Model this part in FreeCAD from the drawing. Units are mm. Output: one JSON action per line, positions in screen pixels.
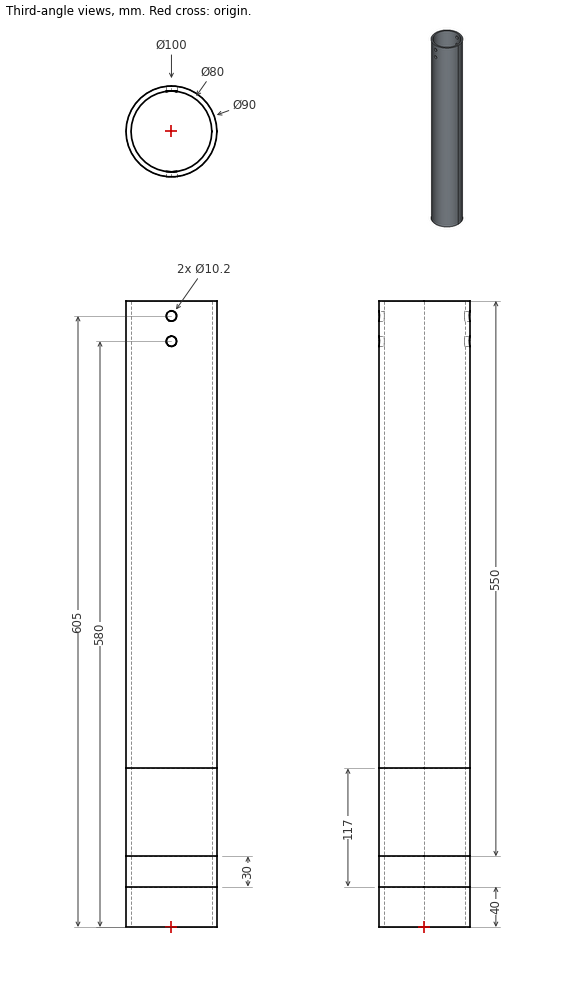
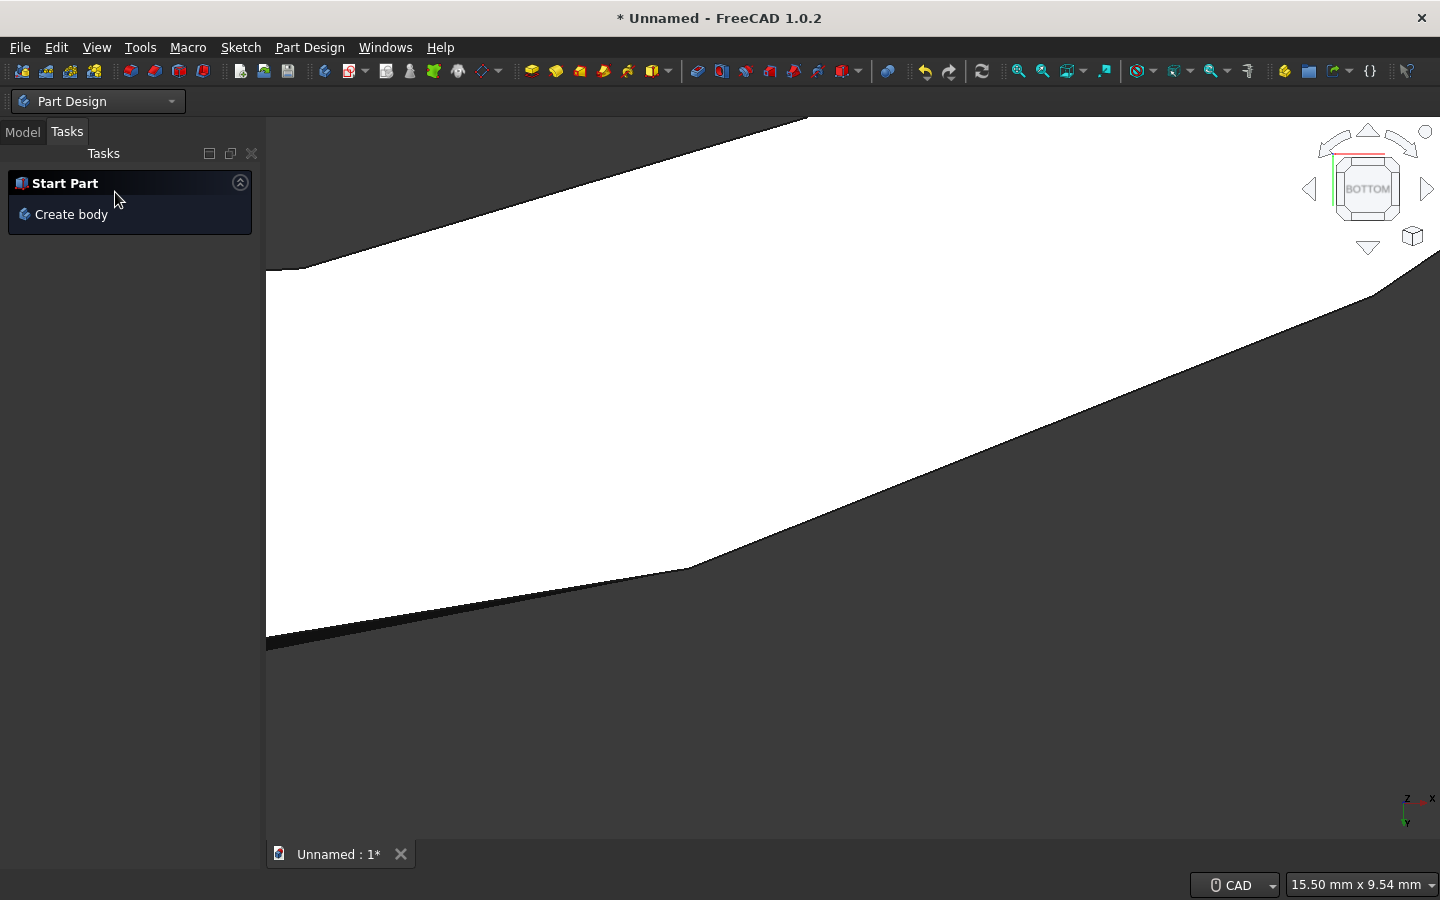
{"action": "key", "text": "0"}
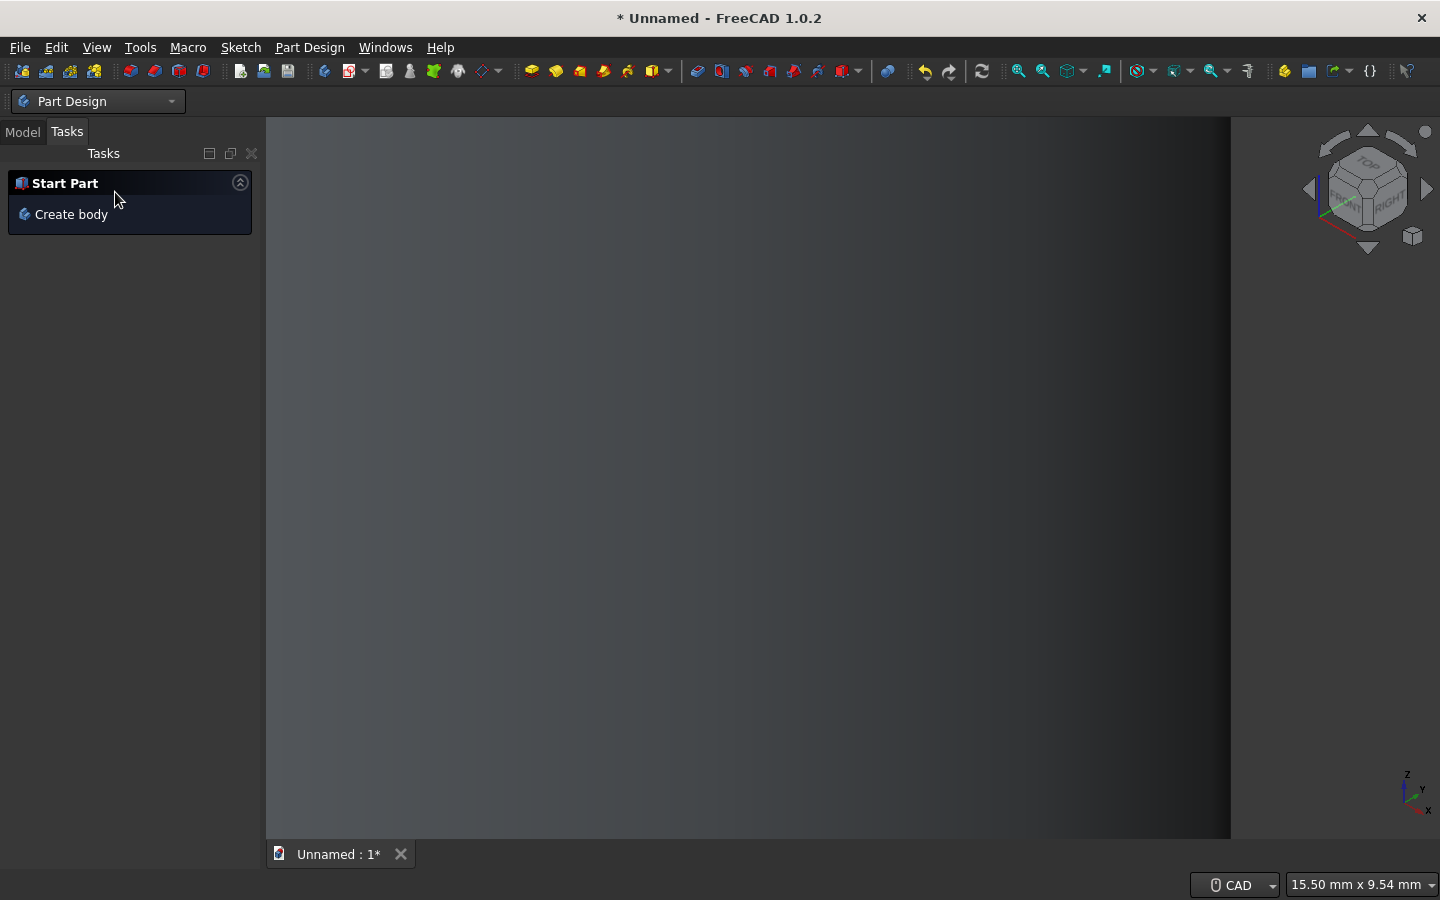
{"action": "left_click", "coordinate": [1020, 72]}